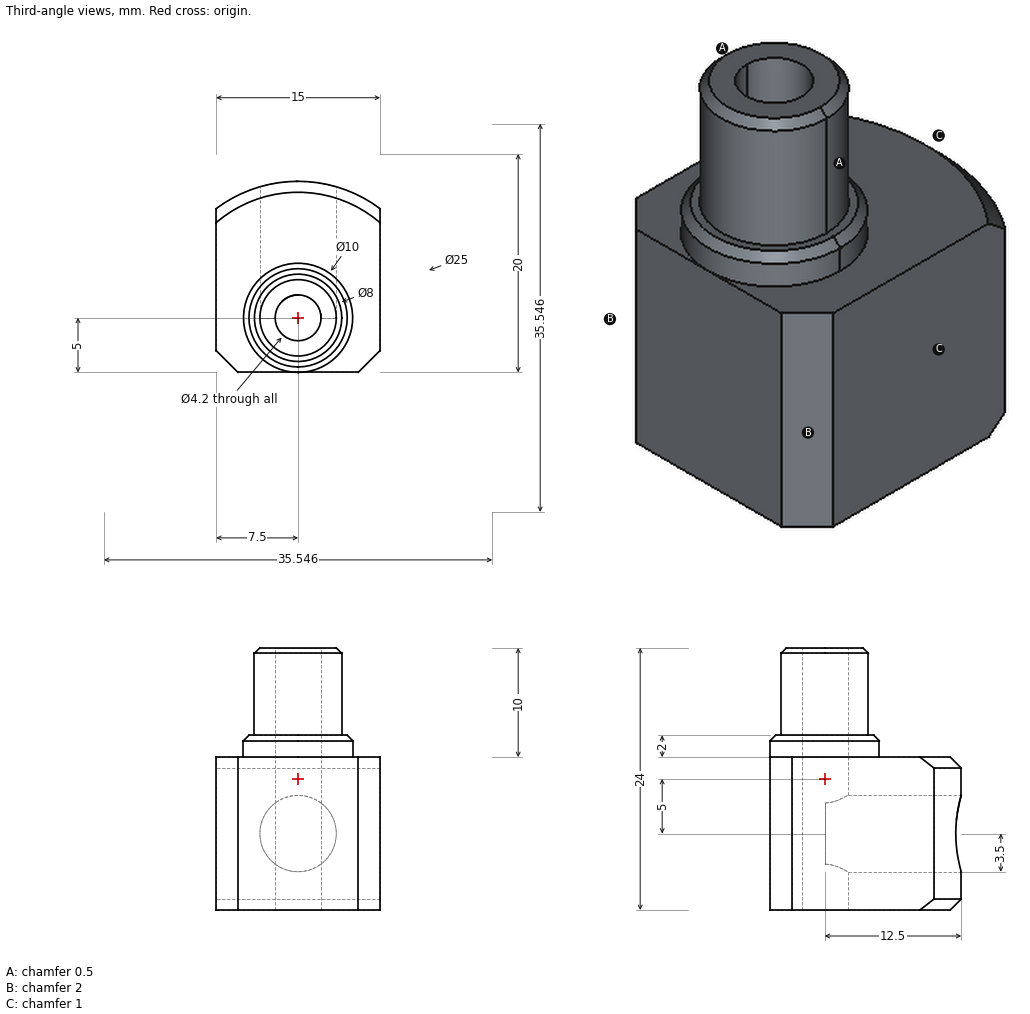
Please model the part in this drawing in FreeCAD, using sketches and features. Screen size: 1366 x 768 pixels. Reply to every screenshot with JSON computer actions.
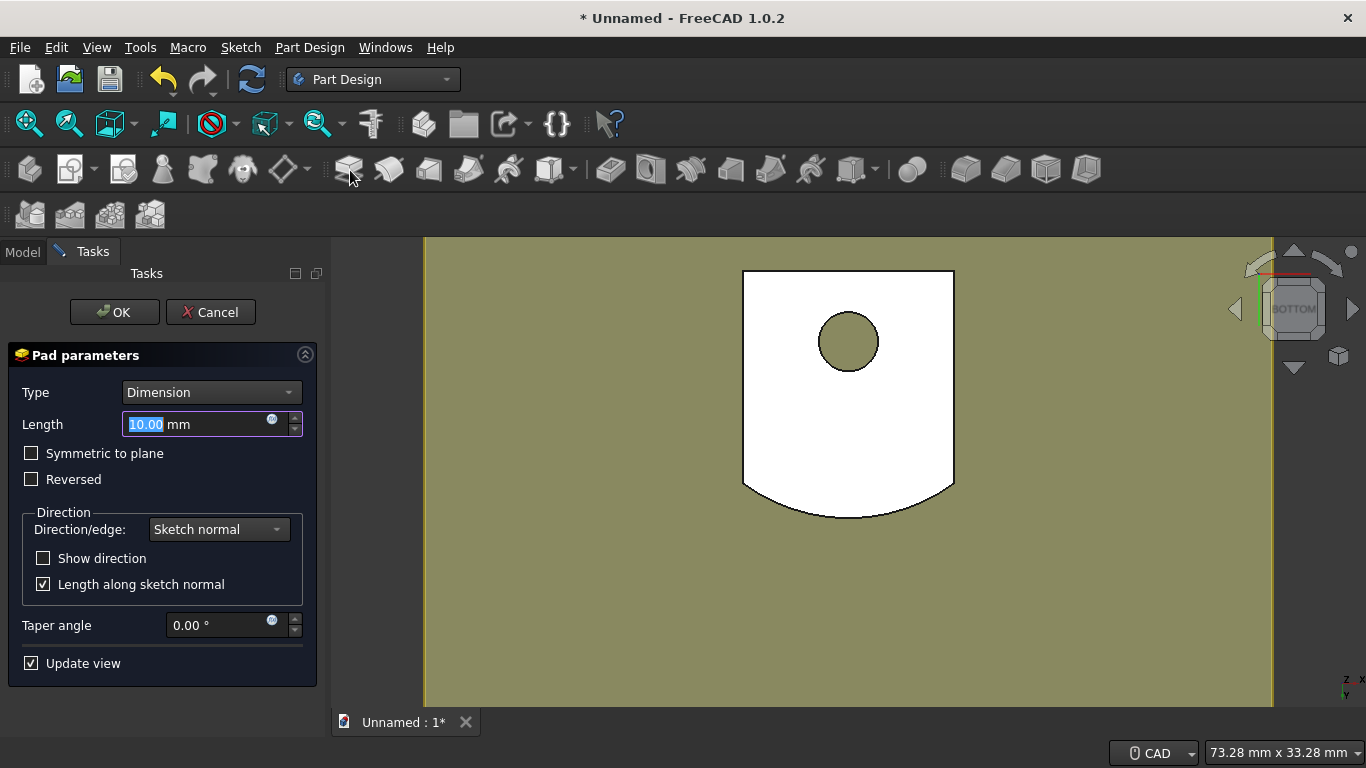
{"action": "type", "text": "2"}
{"action": "key", "text": "Tab"}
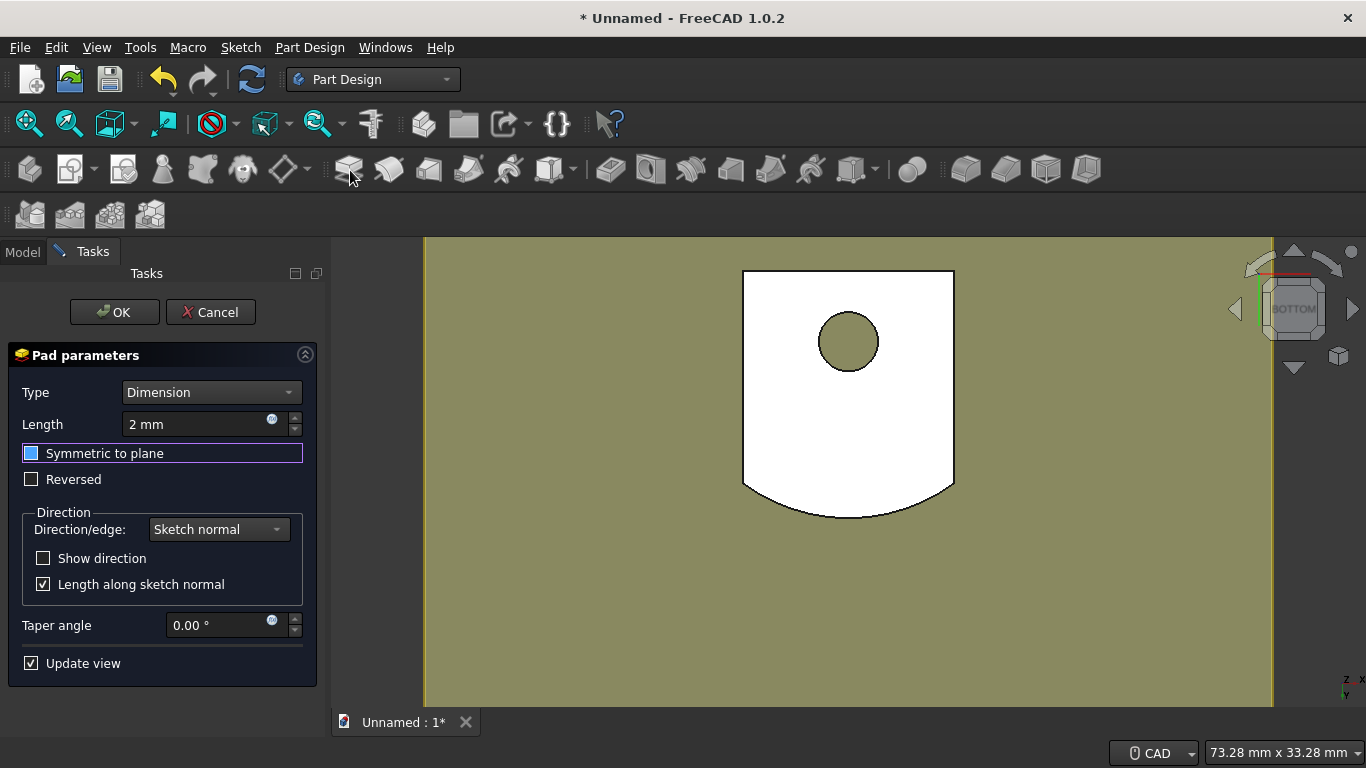
{"action": "left_click", "coordinate": [30, 479]}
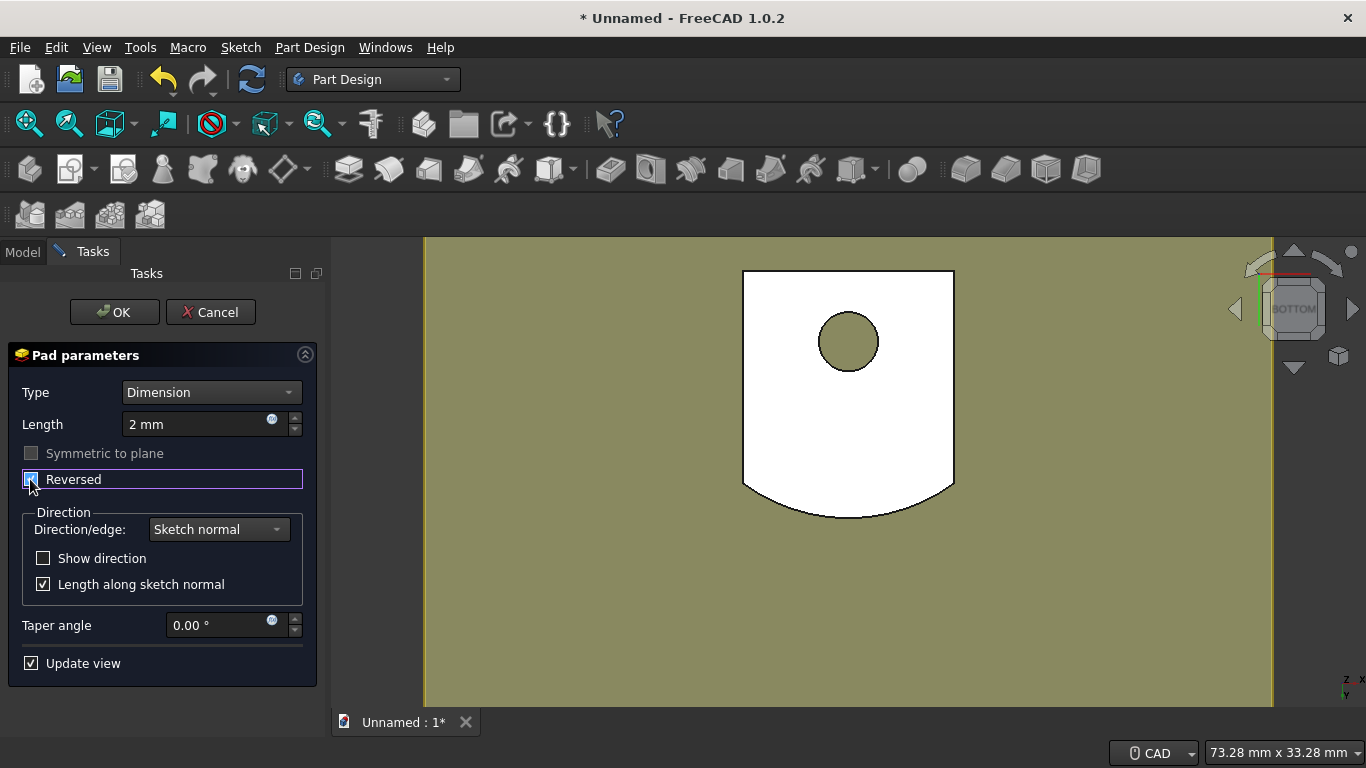
{"action": "left_click", "coordinate": [115, 312]}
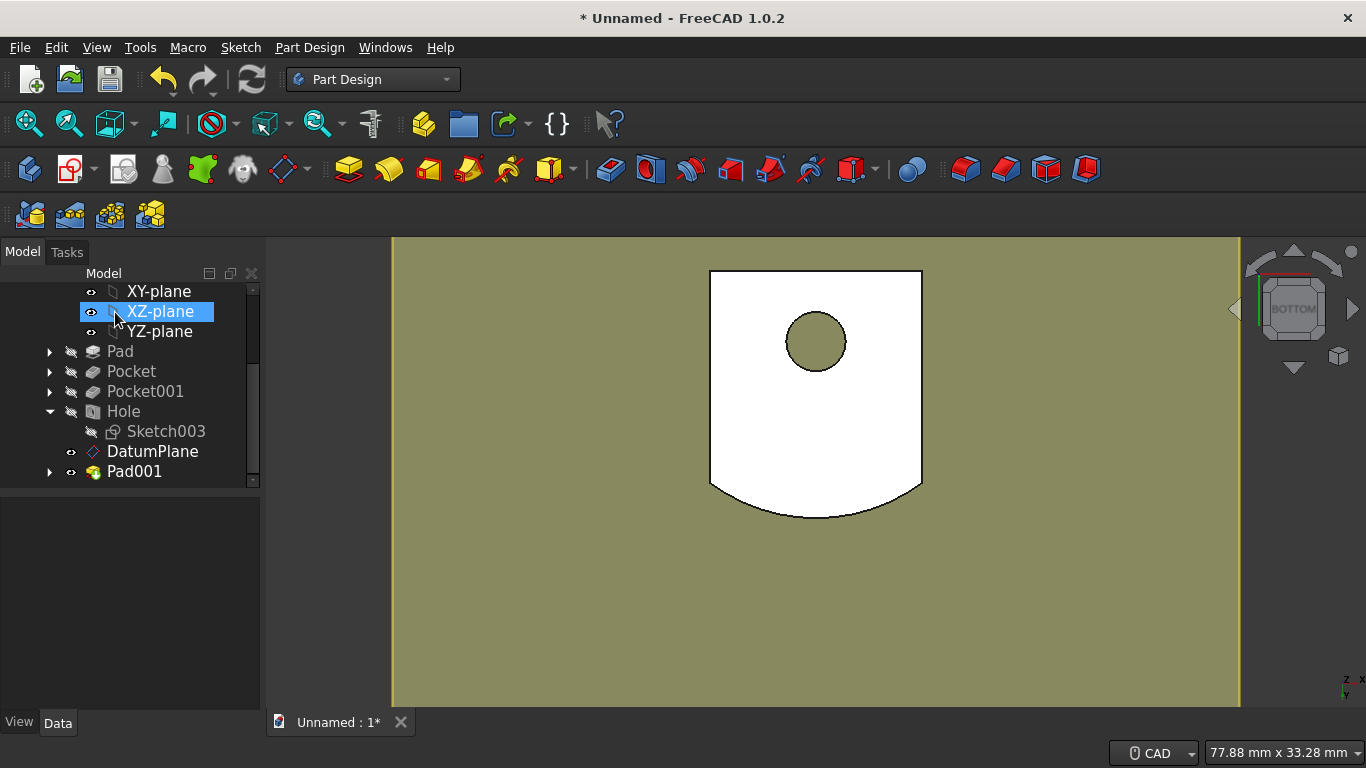
{"action": "left_click", "coordinate": [116, 452]}
{"action": "key", "text": "space"}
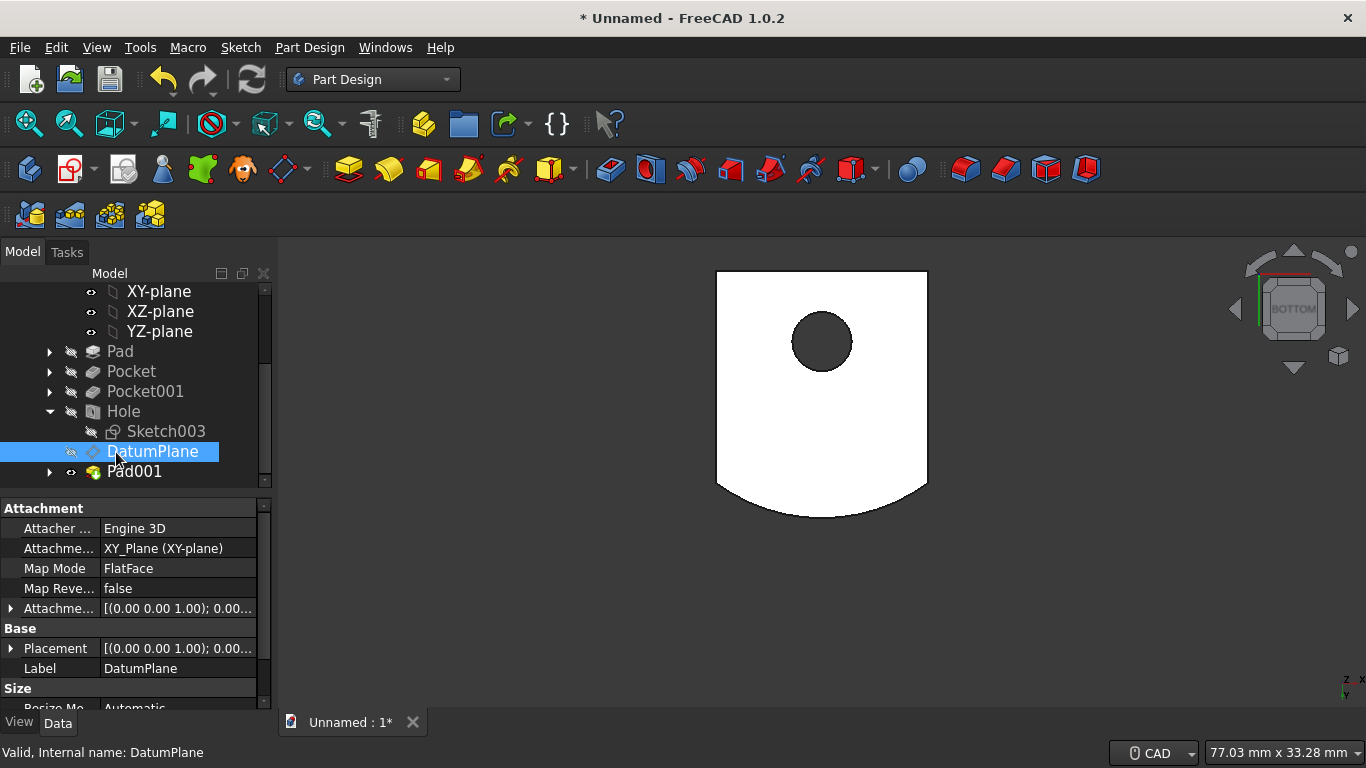
{"action": "left_click", "coordinate": [318, 667]}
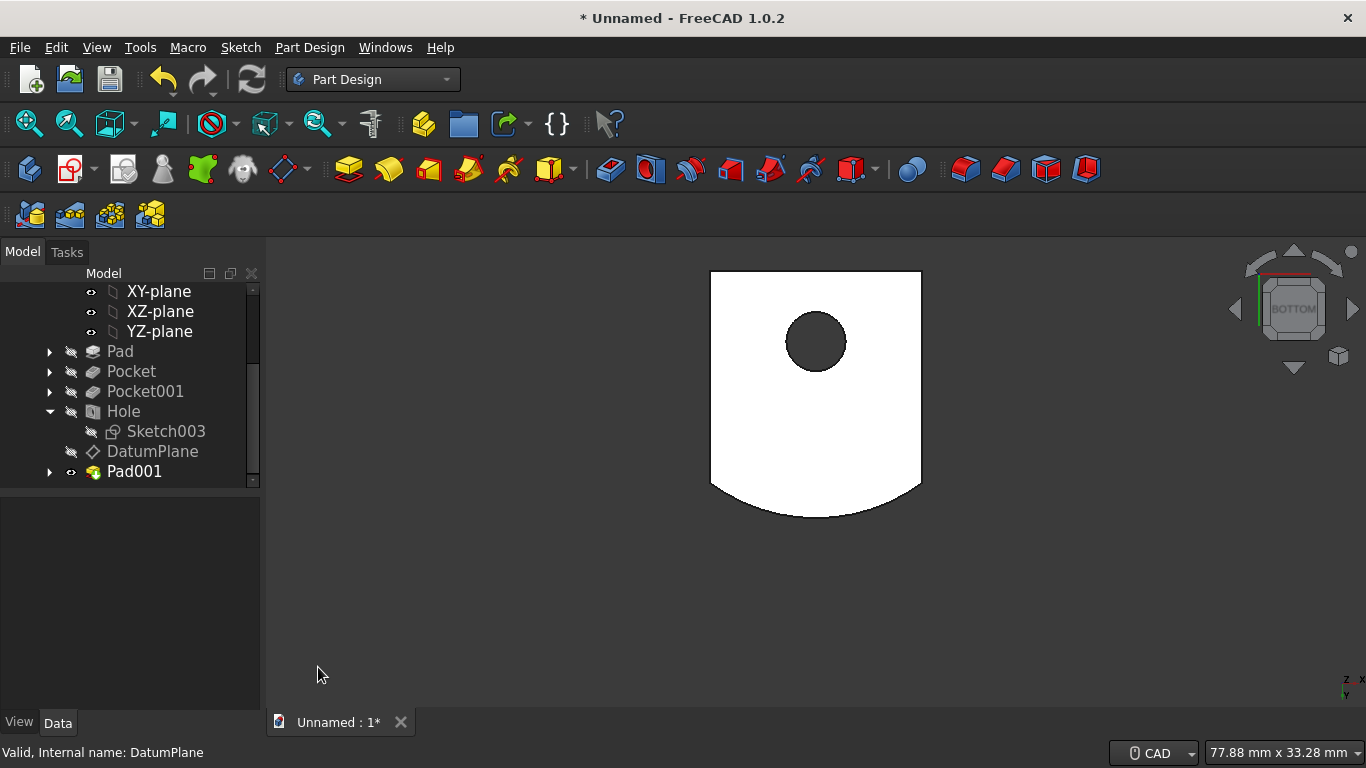
{"action": "left_click", "coordinate": [70, 170]}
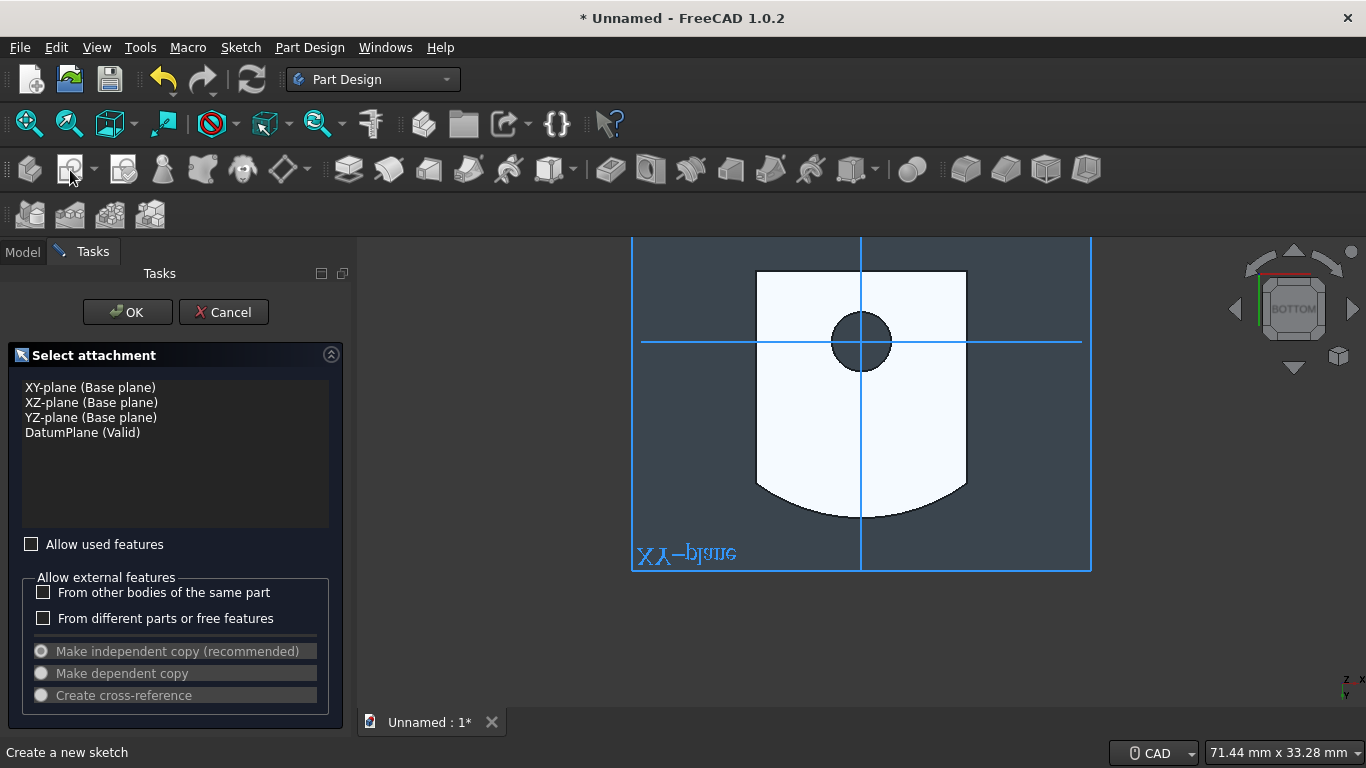
{"action": "left_click", "coordinate": [82, 418]}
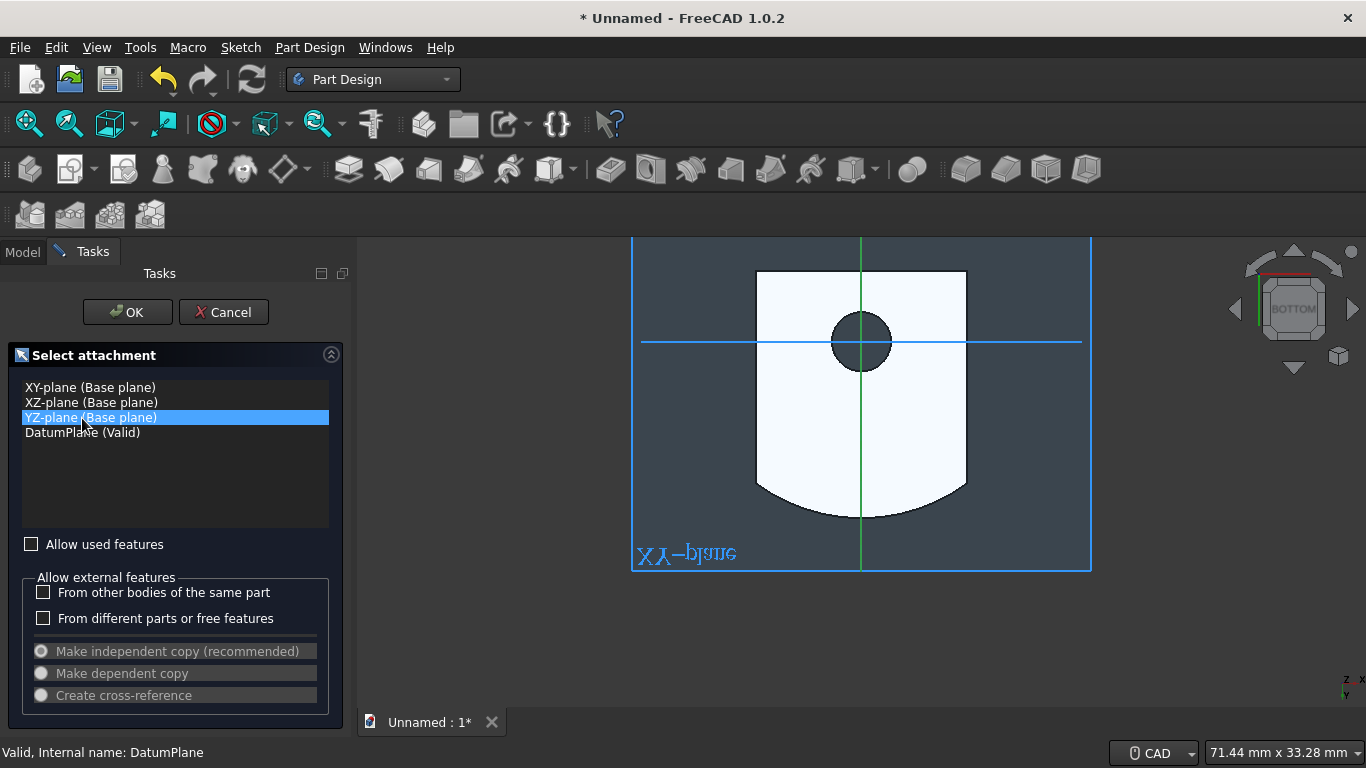
{"action": "left_click", "coordinate": [128, 312]}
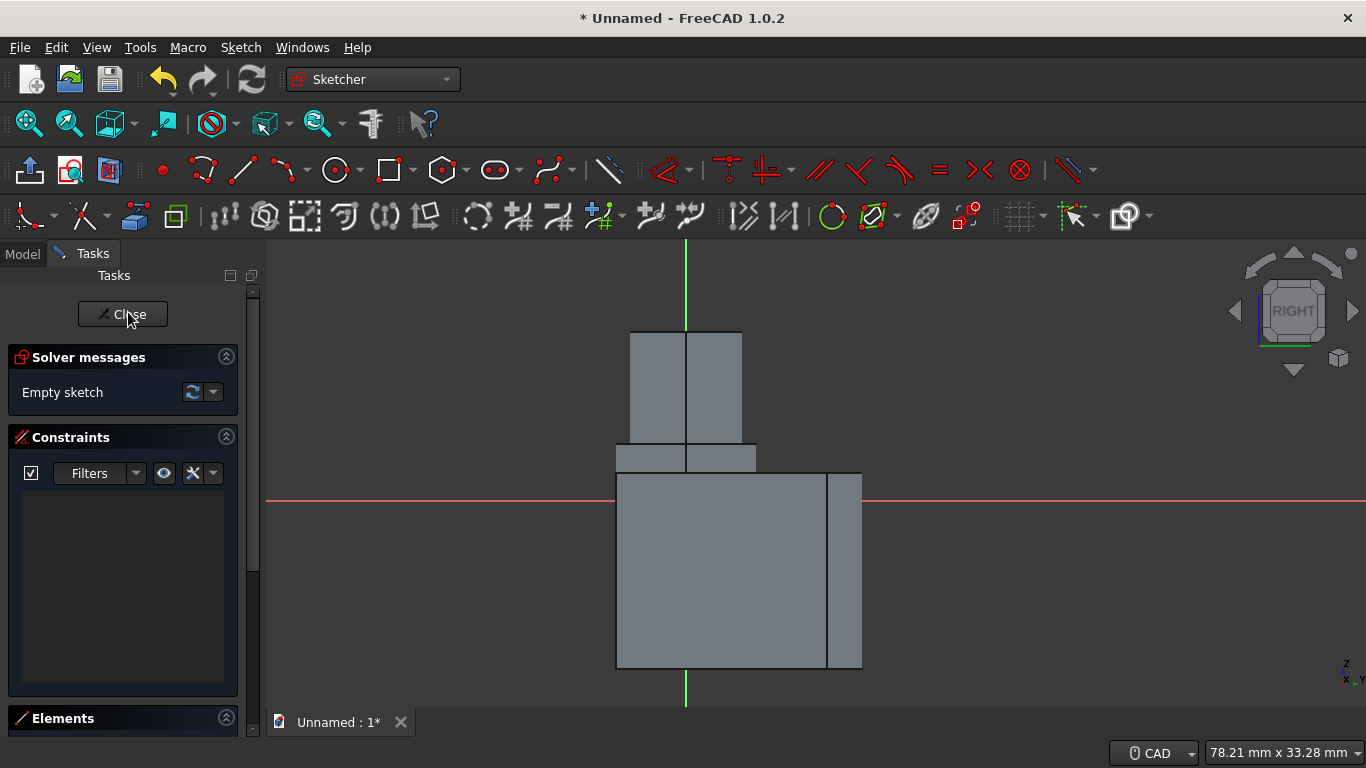
{"action": "left_click", "coordinate": [110, 170]}